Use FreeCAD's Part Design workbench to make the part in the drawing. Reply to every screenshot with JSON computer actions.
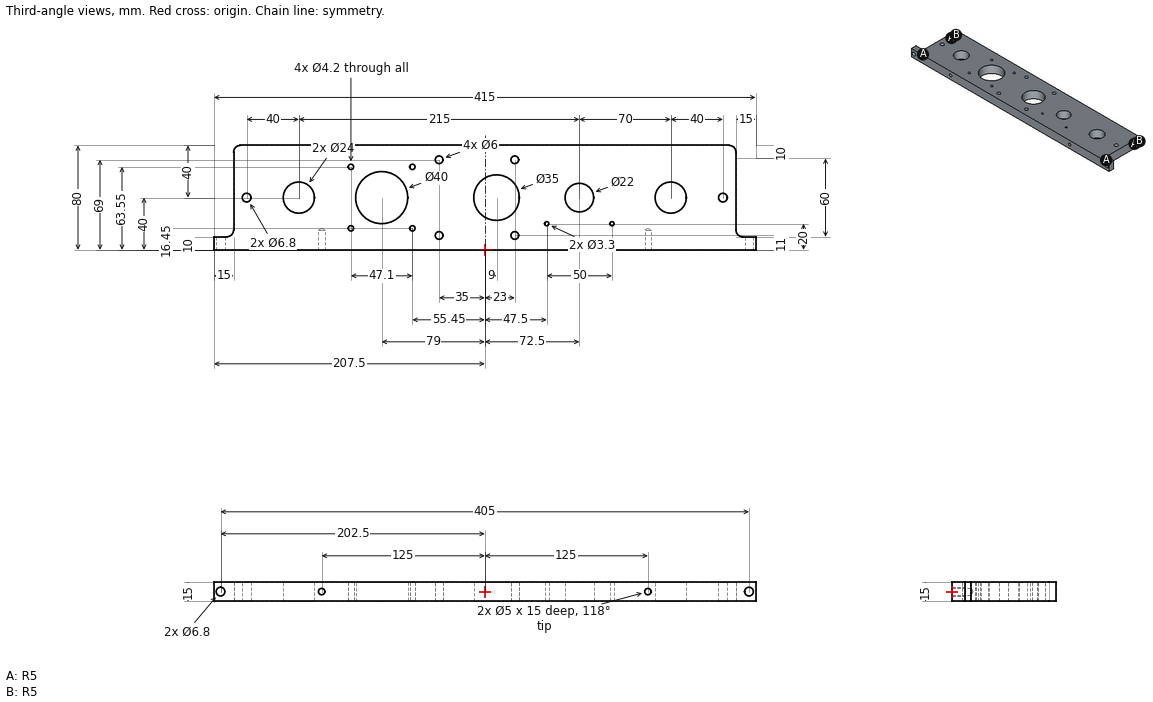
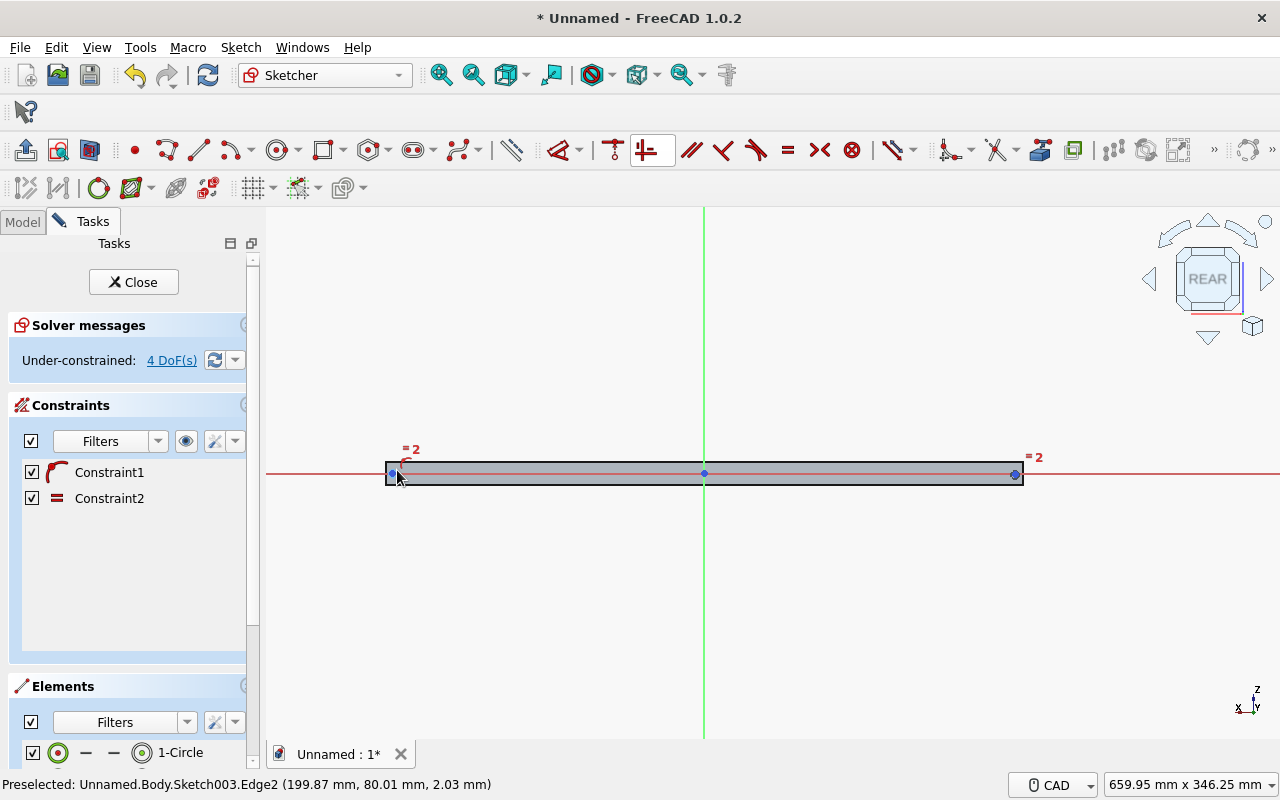
{"action": "left_click", "coordinate": [1015, 475]}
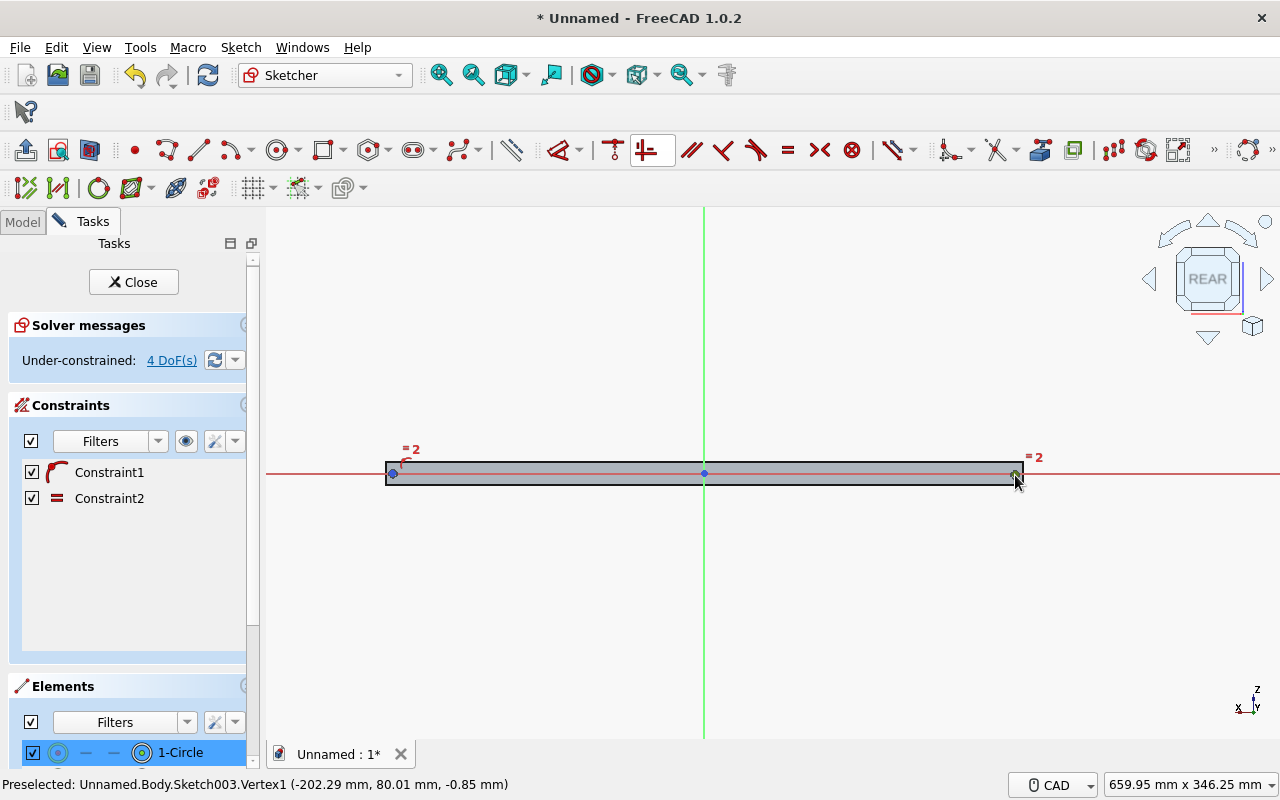
{"action": "left_click", "coordinate": [353, 474]}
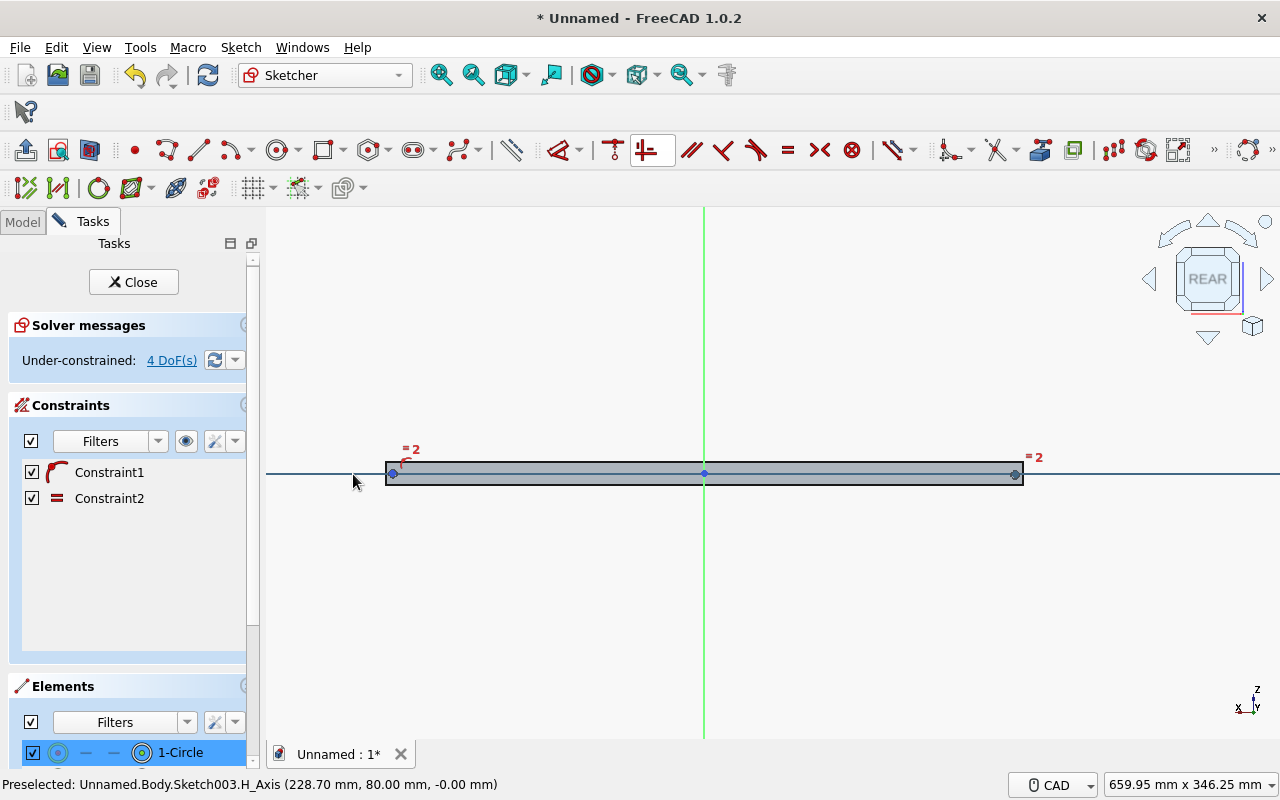
{"action": "left_click", "coordinate": [614, 150]}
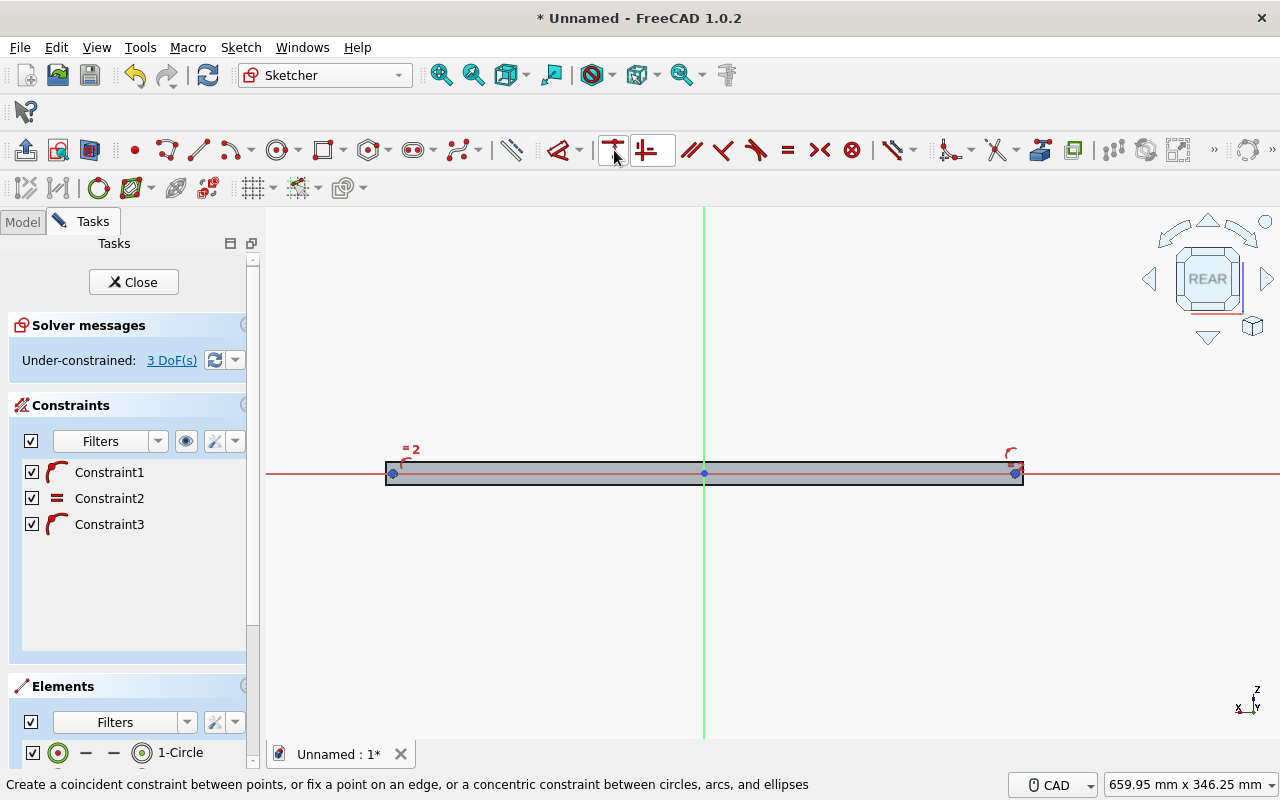
{"action": "left_click", "coordinate": [558, 150]}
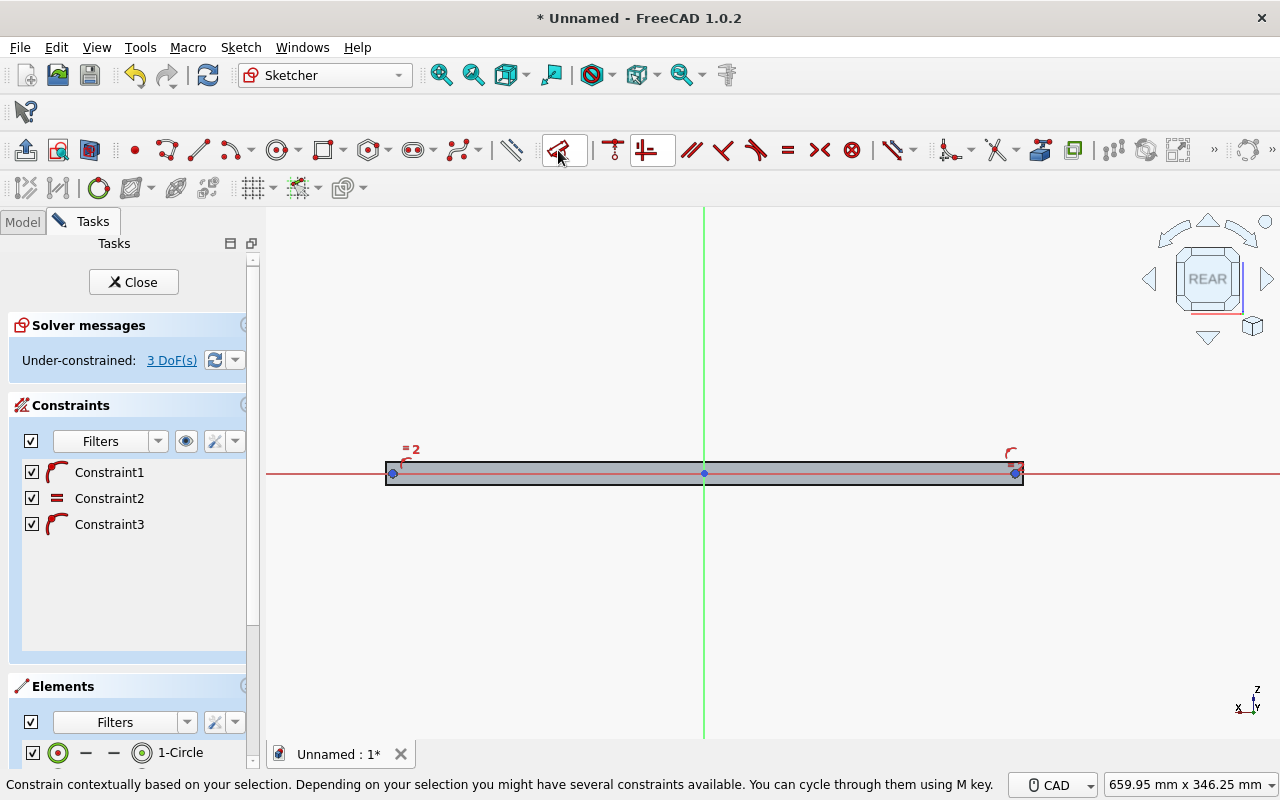
{"action": "scroll", "coordinate": [1018, 477], "scroll_direction": "up", "scroll_amount": 7}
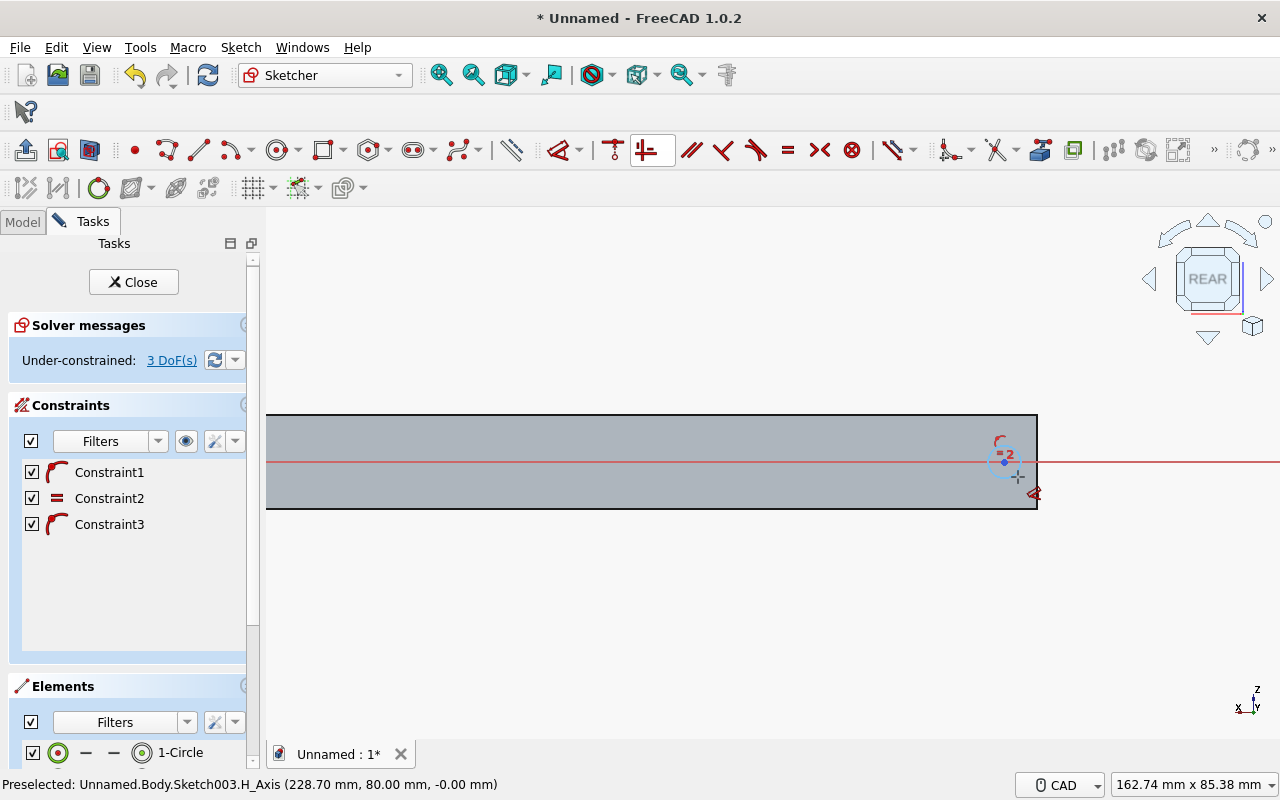
{"action": "left_click", "coordinate": [1016, 473]}
{"action": "left_click", "coordinate": [1039, 495]}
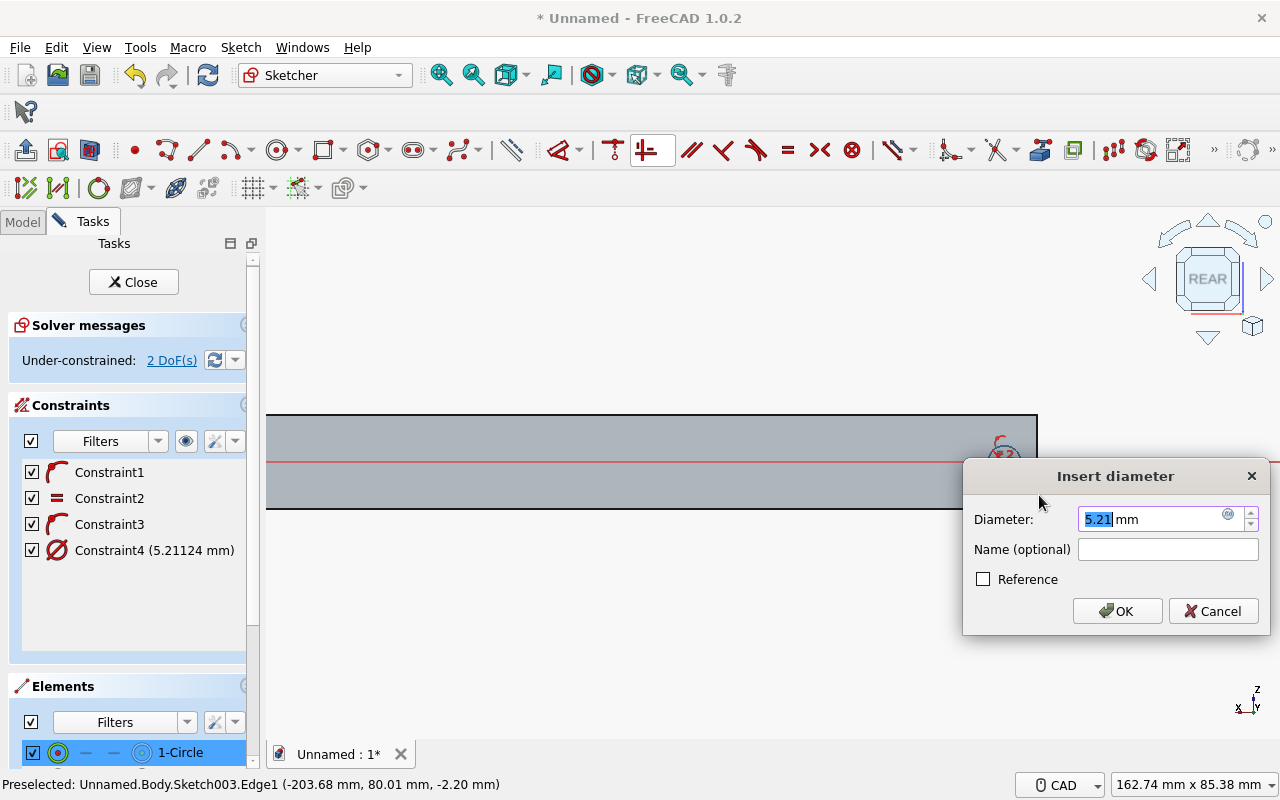
{"action": "type", "text": "6.8"}
{"action": "key", "text": "Return"}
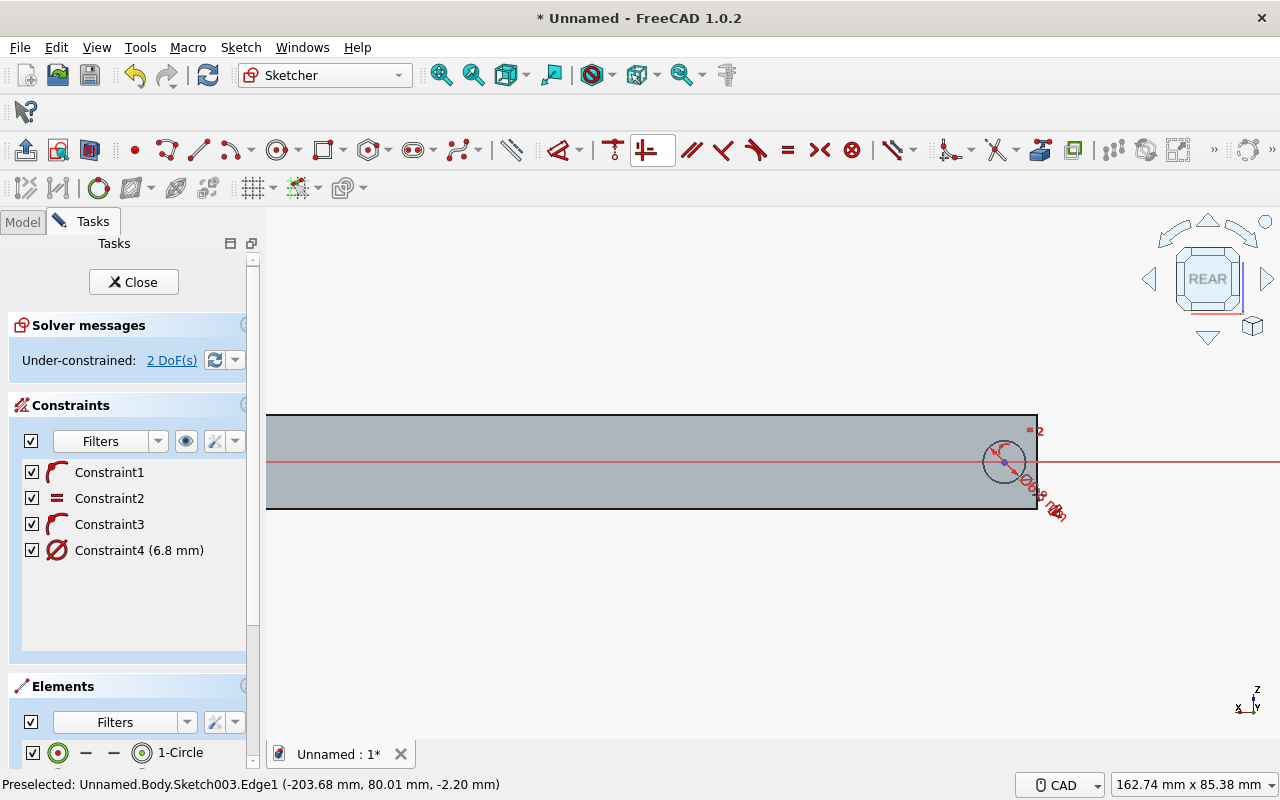
{"action": "scroll", "coordinate": [1019, 477], "scroll_direction": "down", "scroll_amount": 7}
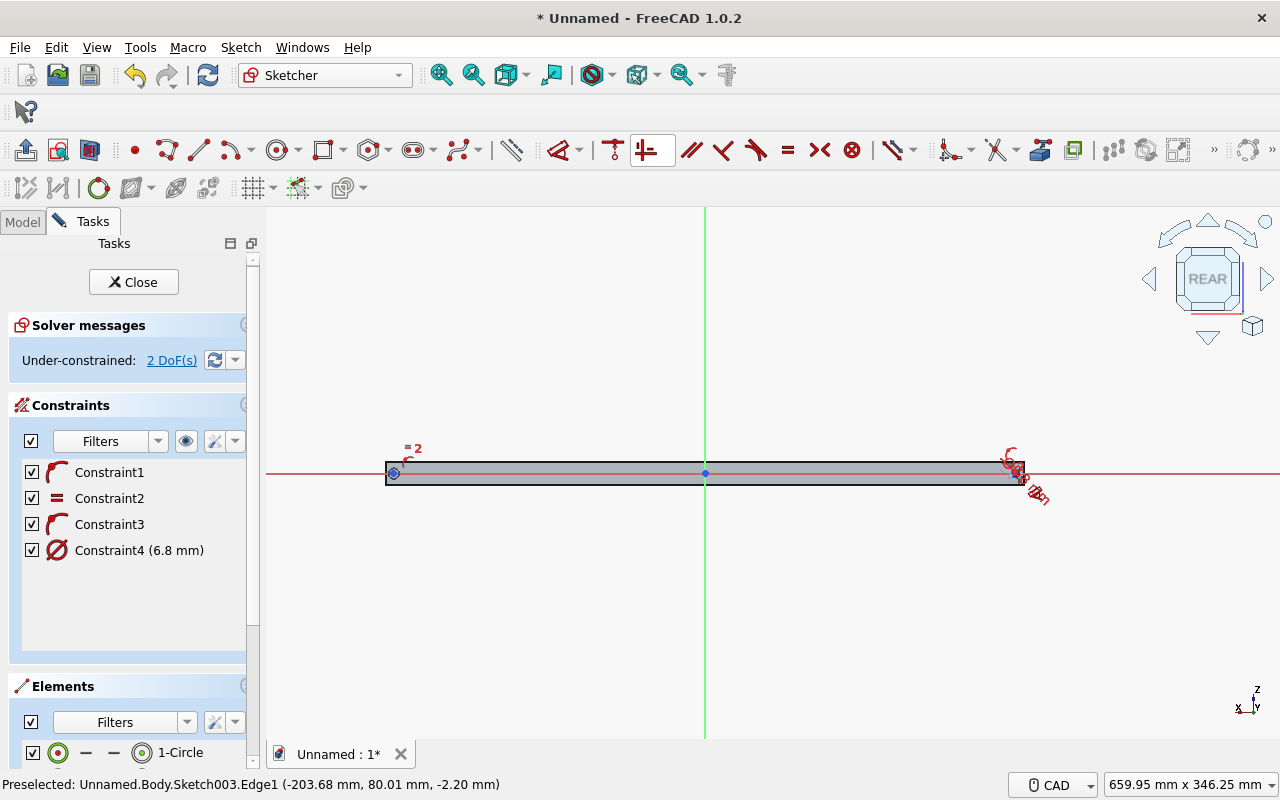
{"action": "left_click", "coordinate": [1016, 474]}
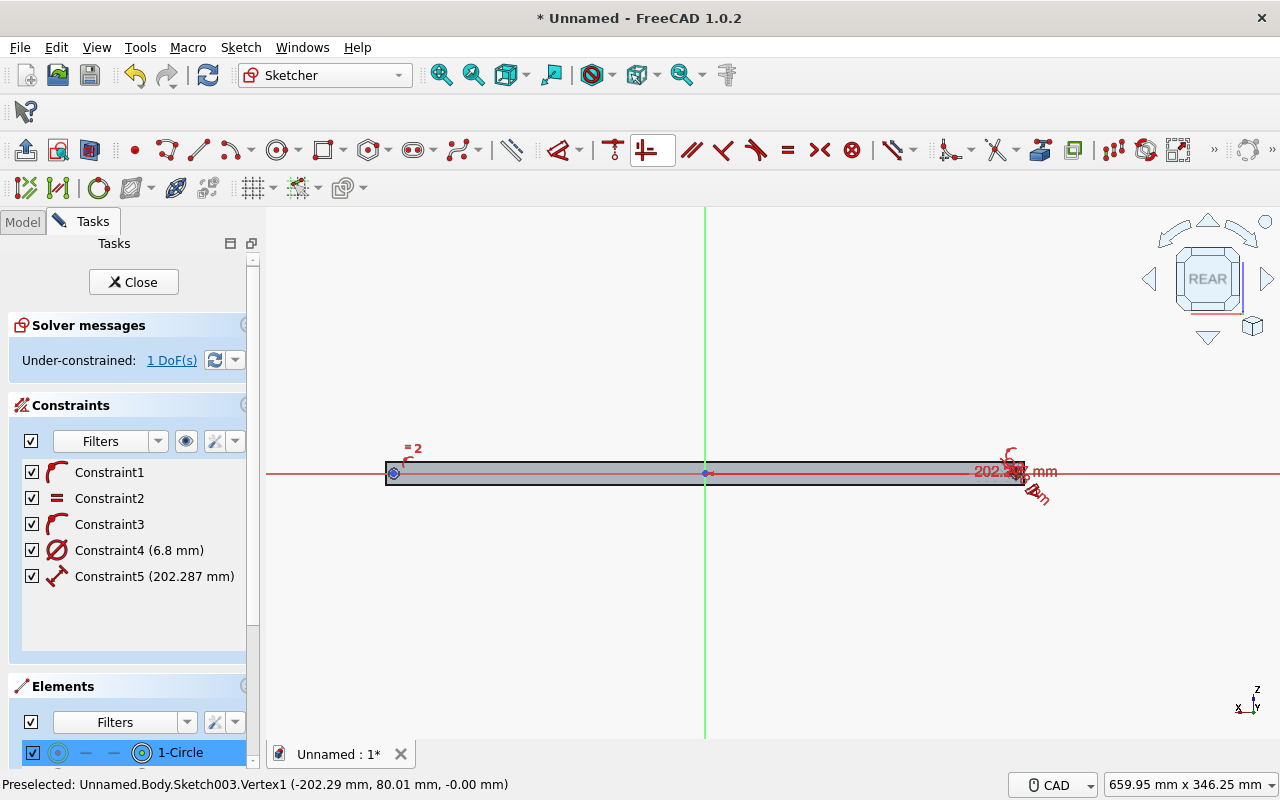
{"action": "left_click", "coordinate": [394, 474]}
{"action": "left_click", "coordinate": [562, 508]}